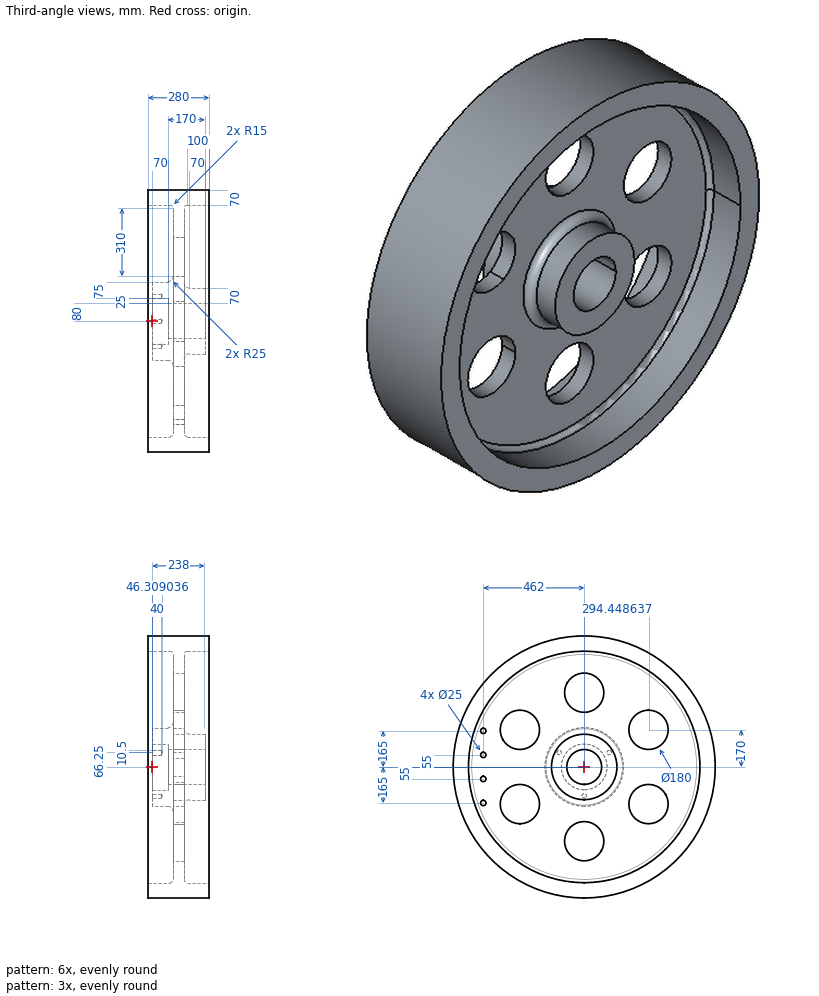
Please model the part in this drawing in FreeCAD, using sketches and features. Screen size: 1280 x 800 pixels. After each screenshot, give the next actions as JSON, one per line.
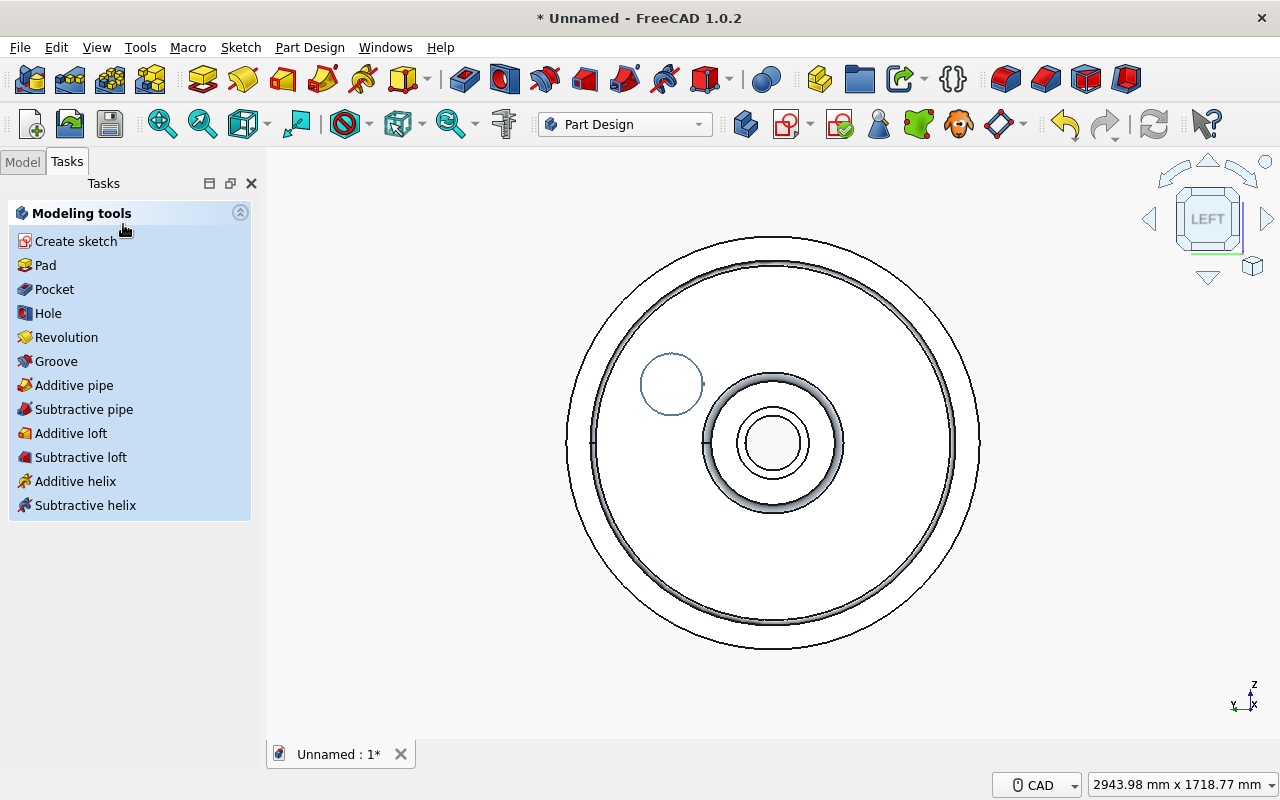
{"action": "left_click", "coordinate": [466, 80]}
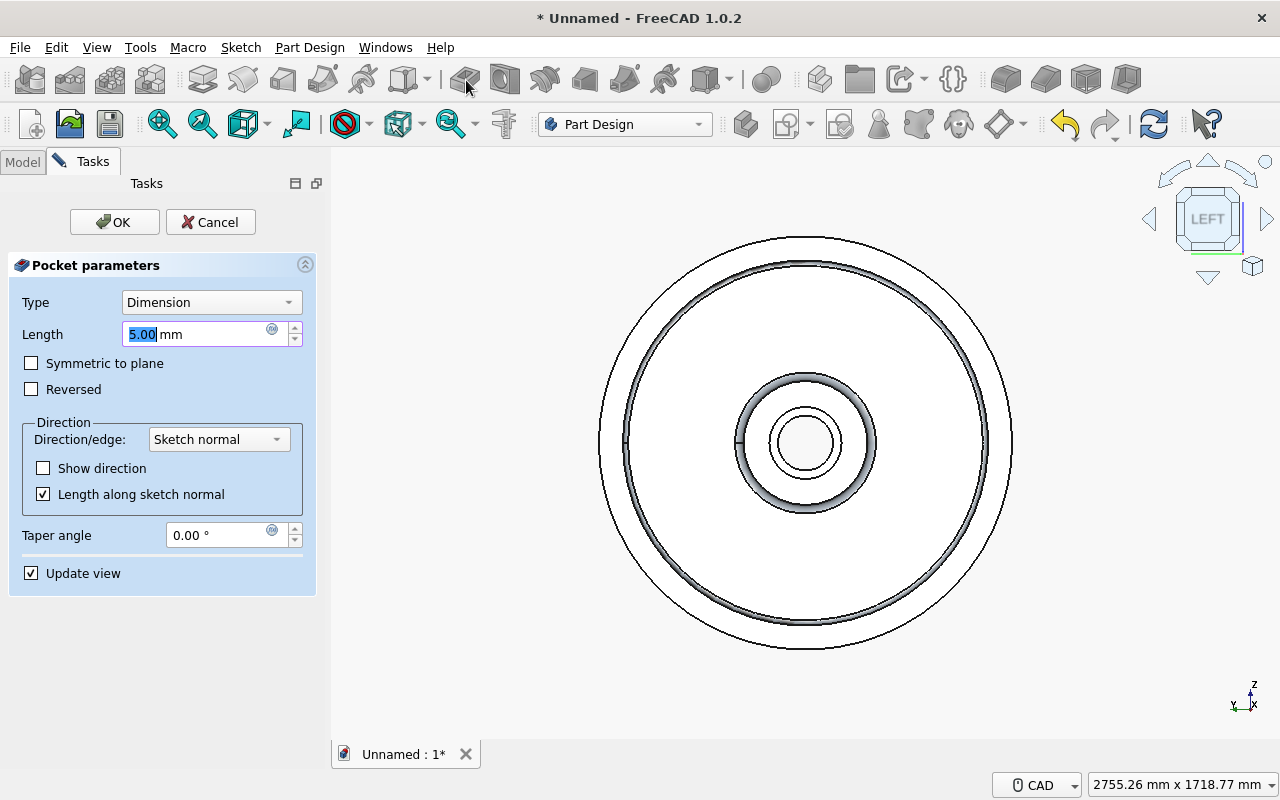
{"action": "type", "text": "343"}
{"action": "key", "text": "Tab"}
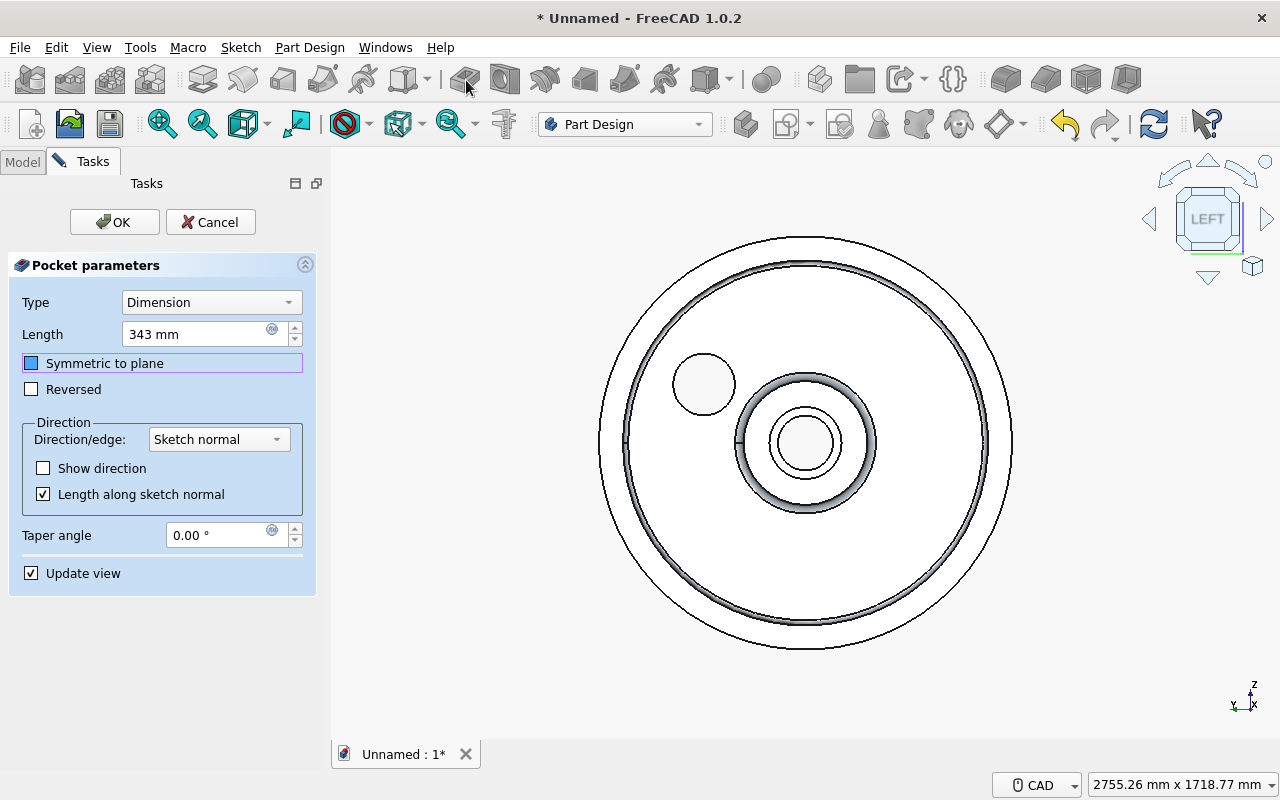
{"action": "left_click", "coordinate": [115, 222]}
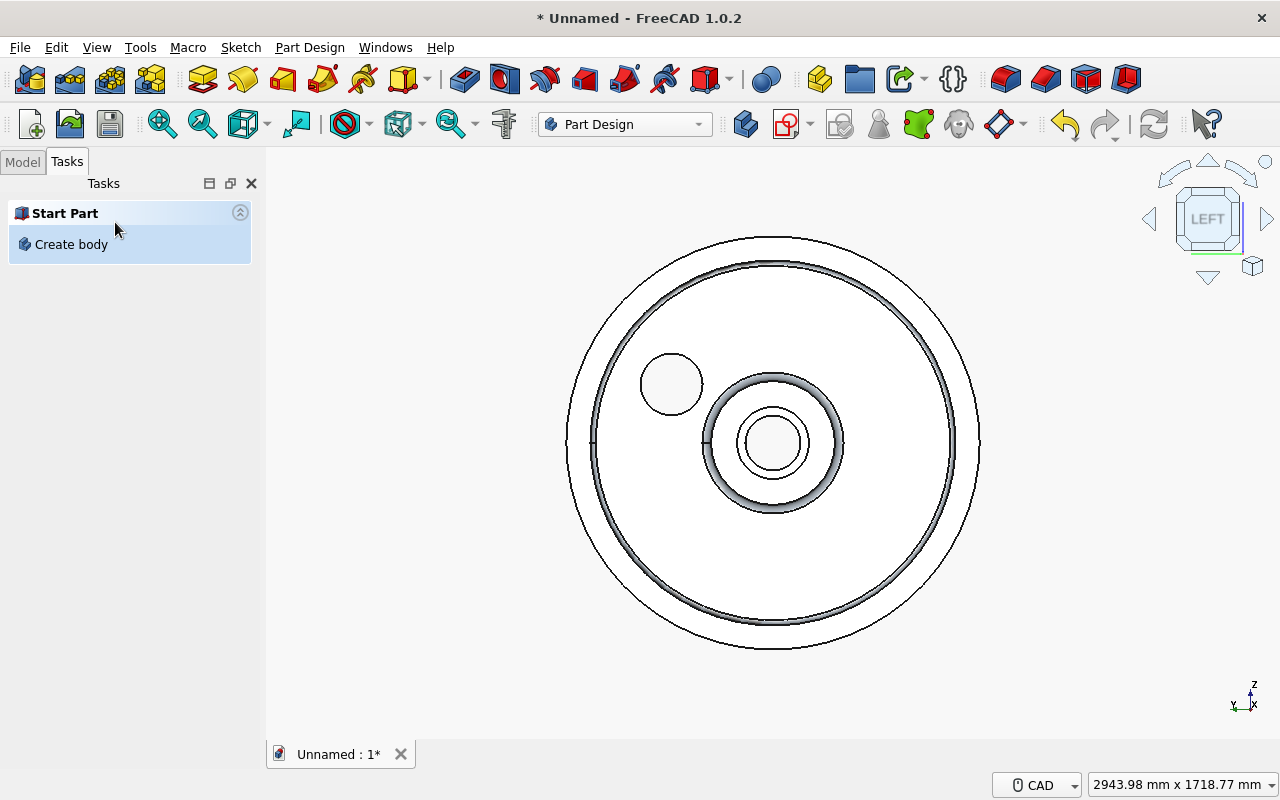
{"action": "left_click", "coordinate": [23, 161]}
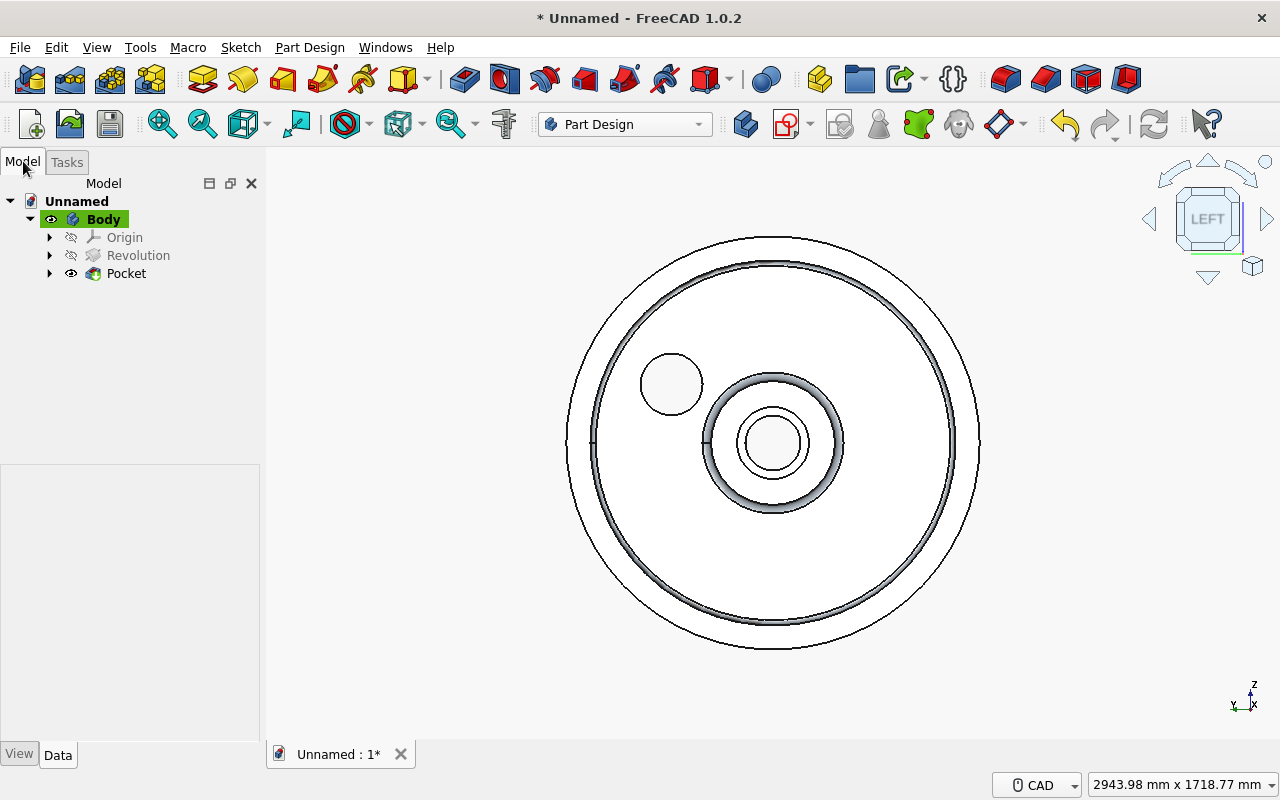
{"action": "left_click", "coordinate": [116, 273]}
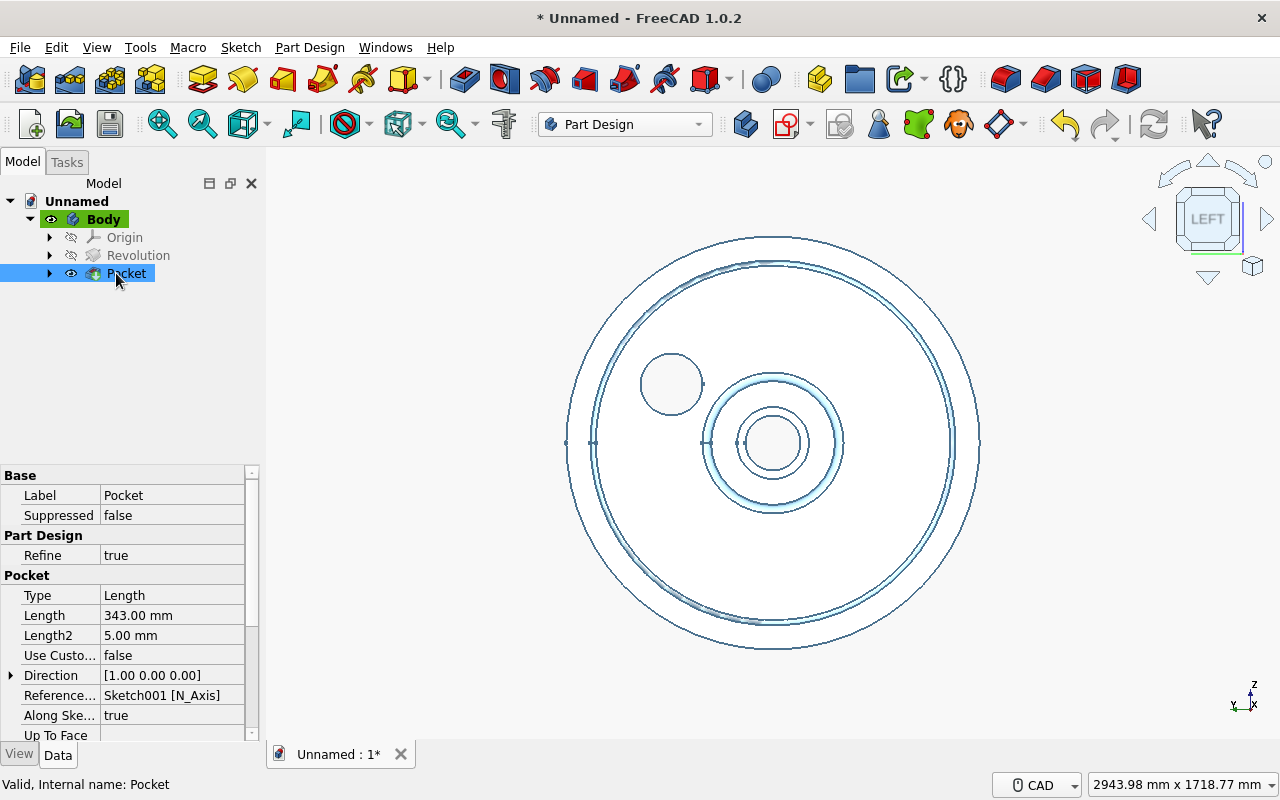
{"action": "left_click", "coordinate": [110, 80]}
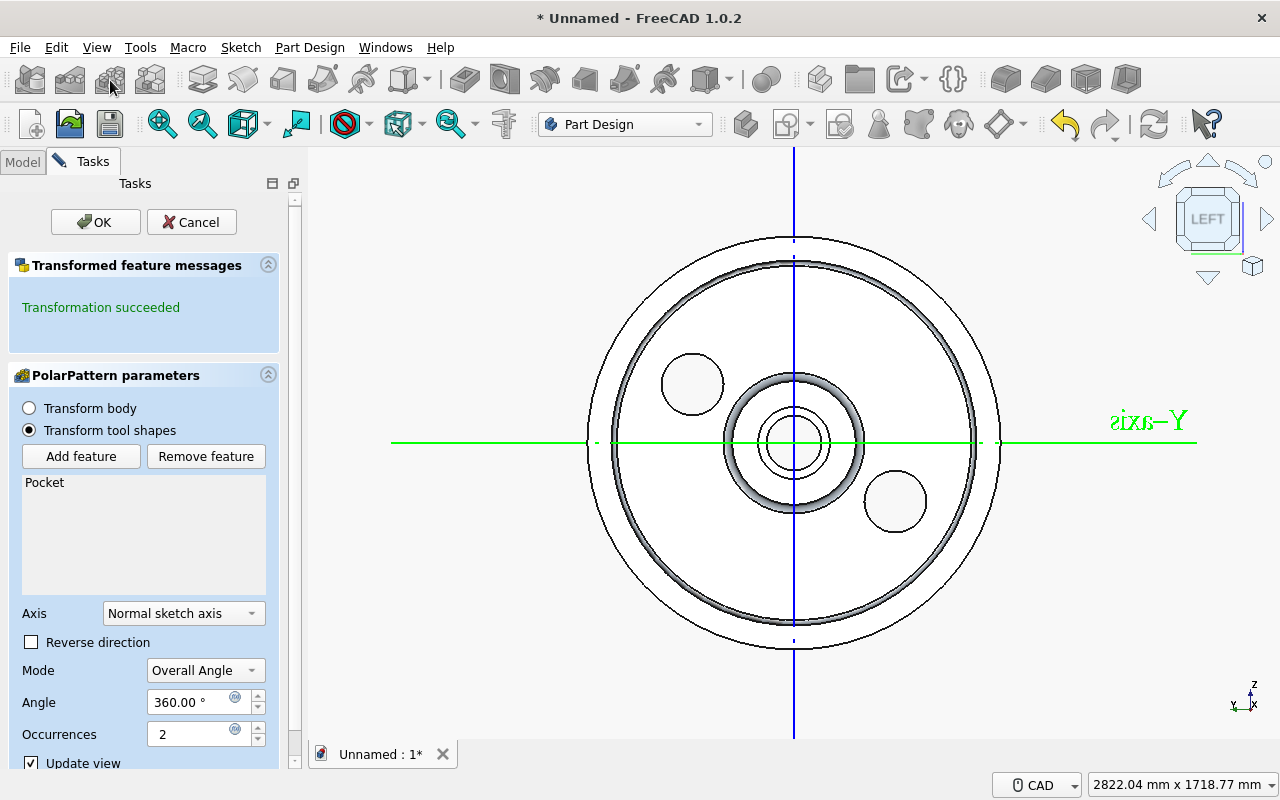
{"action": "left_click", "coordinate": [184, 614]}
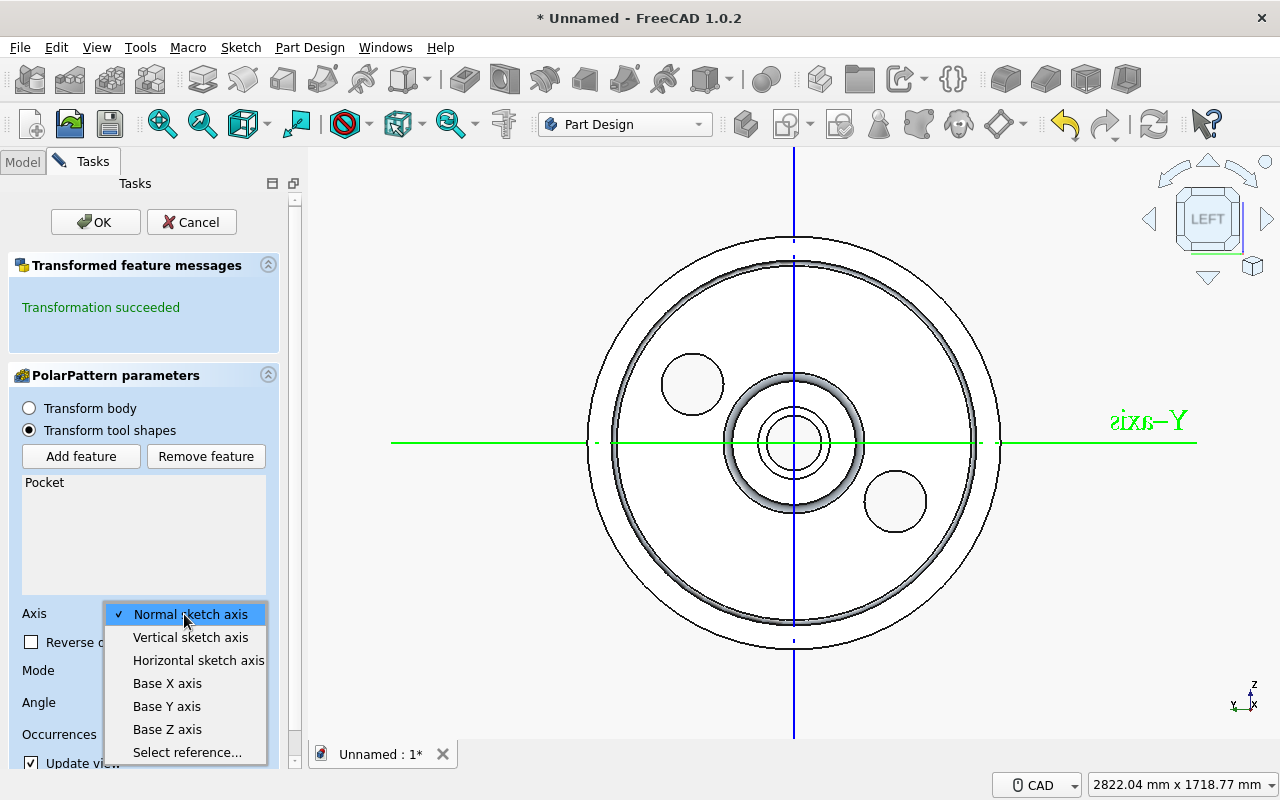
{"action": "left_click", "coordinate": [184, 684]}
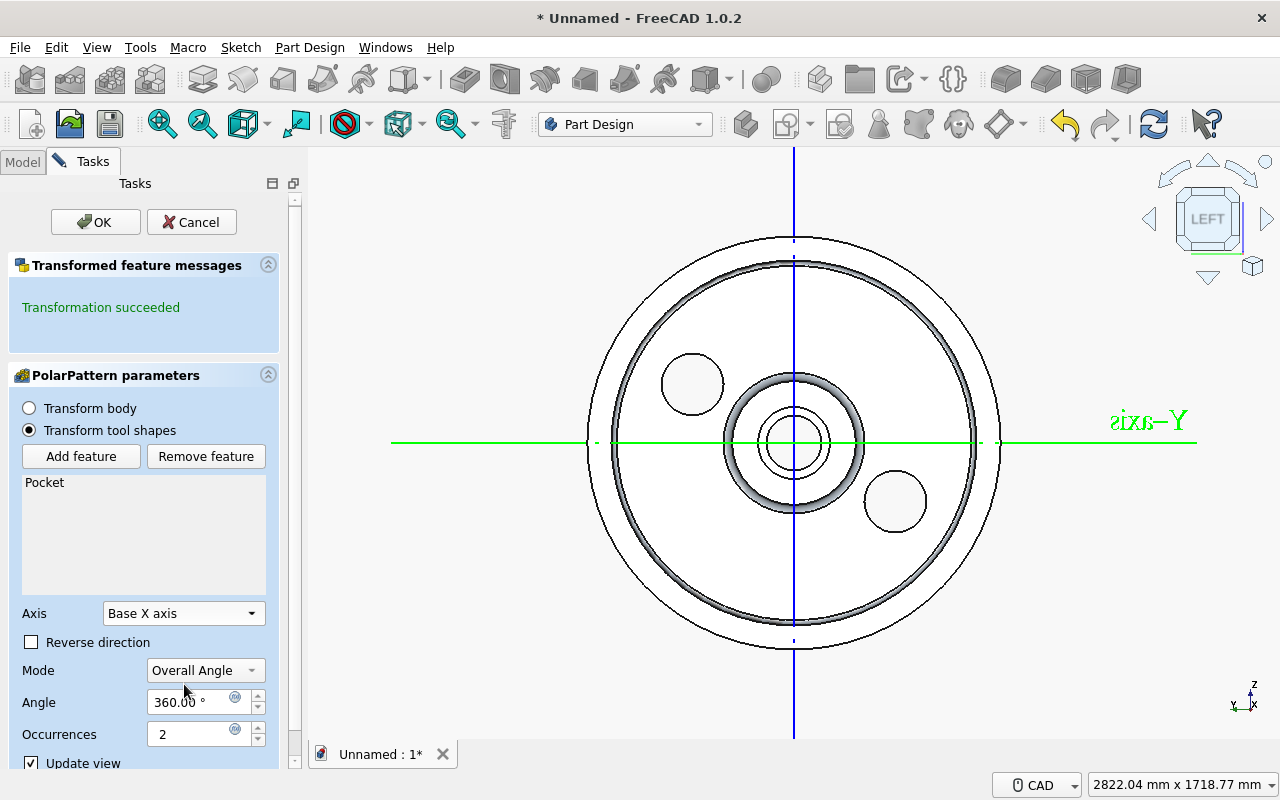
{"action": "triple_click", "coordinate": [198, 734]}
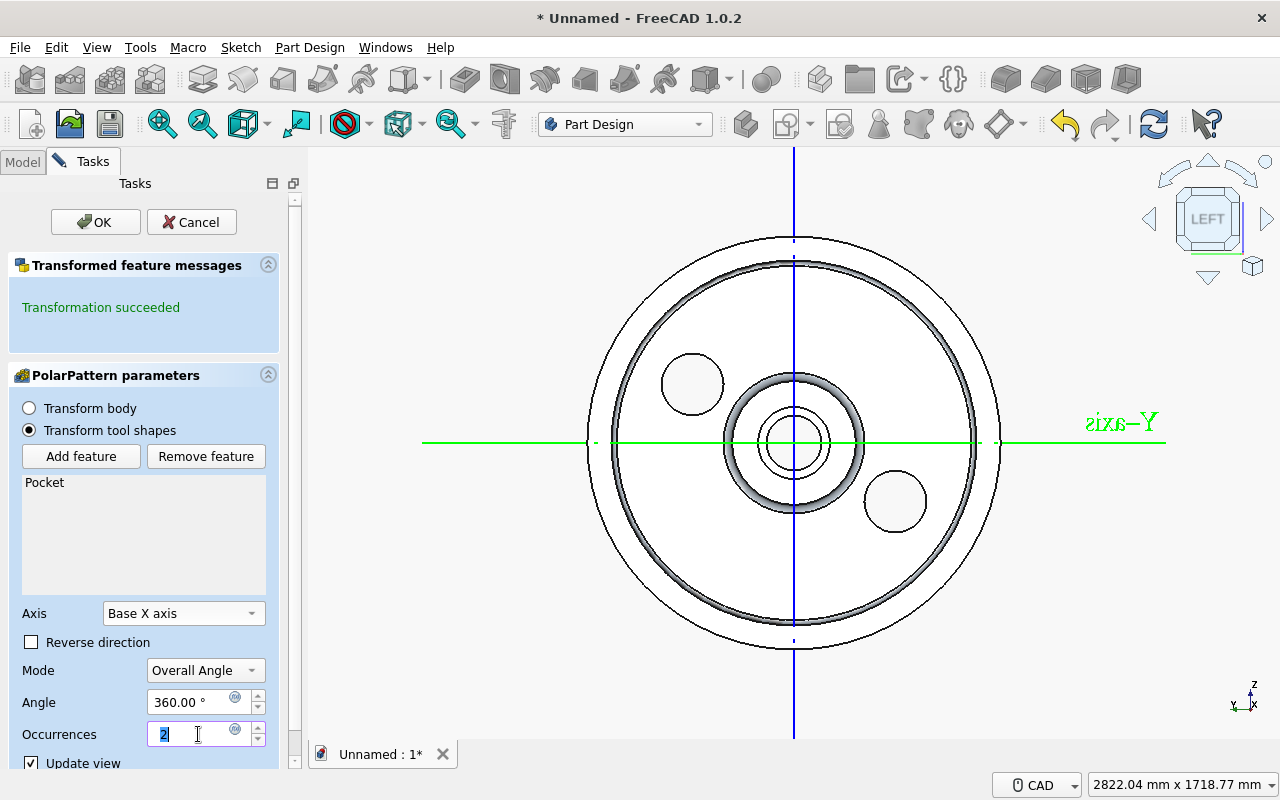
{"action": "type", "text": "6"}
{"action": "key", "text": "Tab"}